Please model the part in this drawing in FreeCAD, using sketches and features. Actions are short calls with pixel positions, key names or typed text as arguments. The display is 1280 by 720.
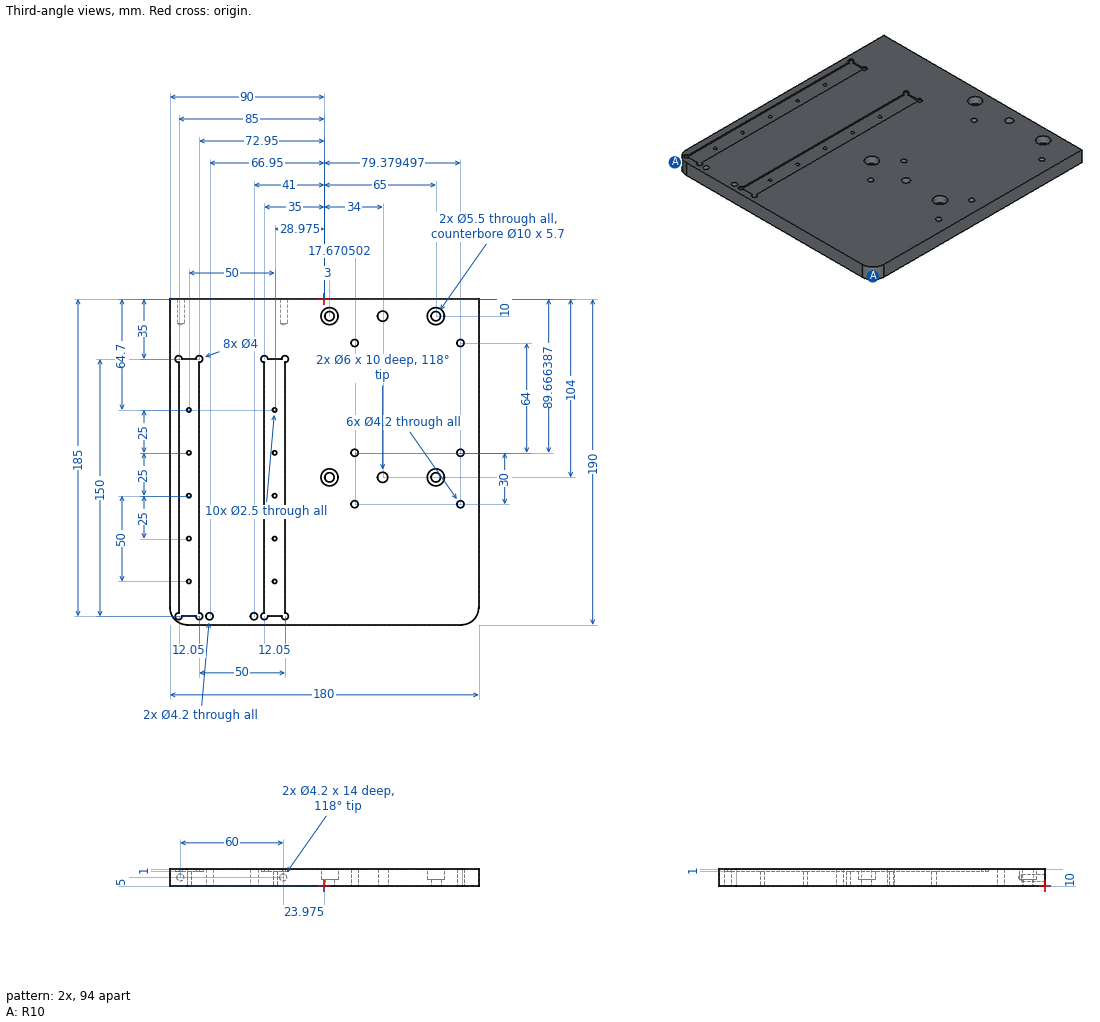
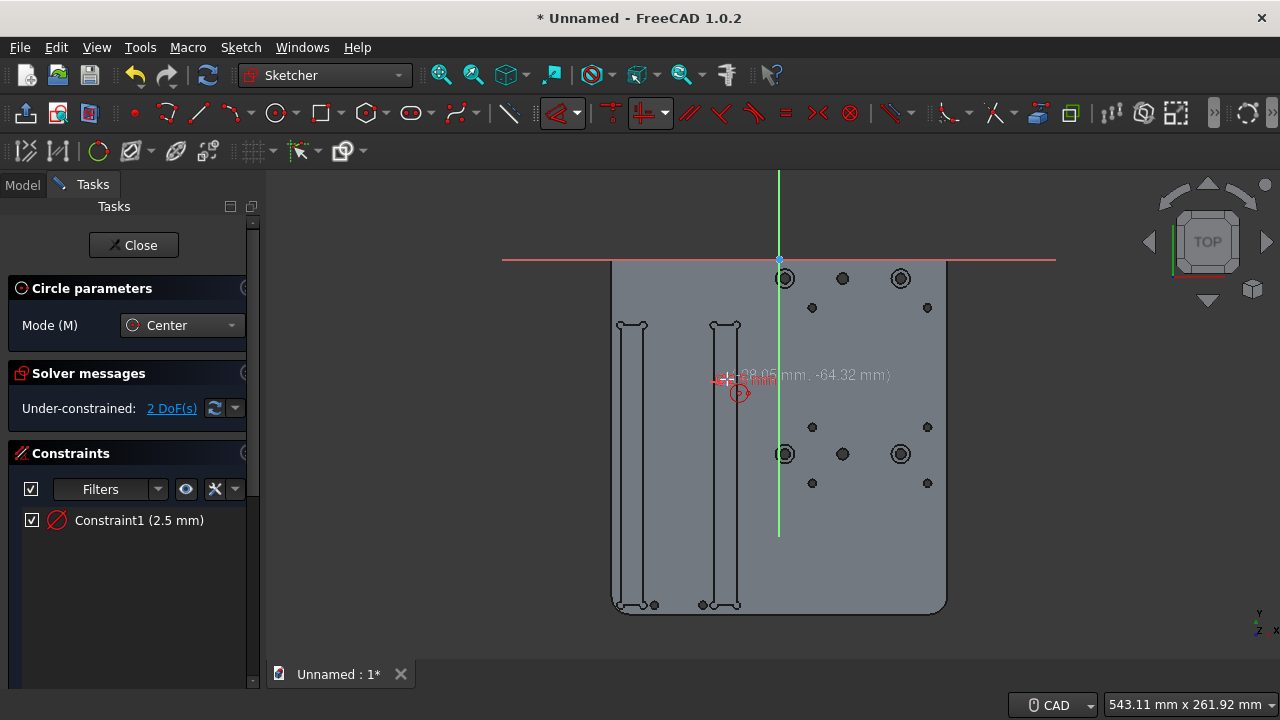
scroll(632, 381, up, 12)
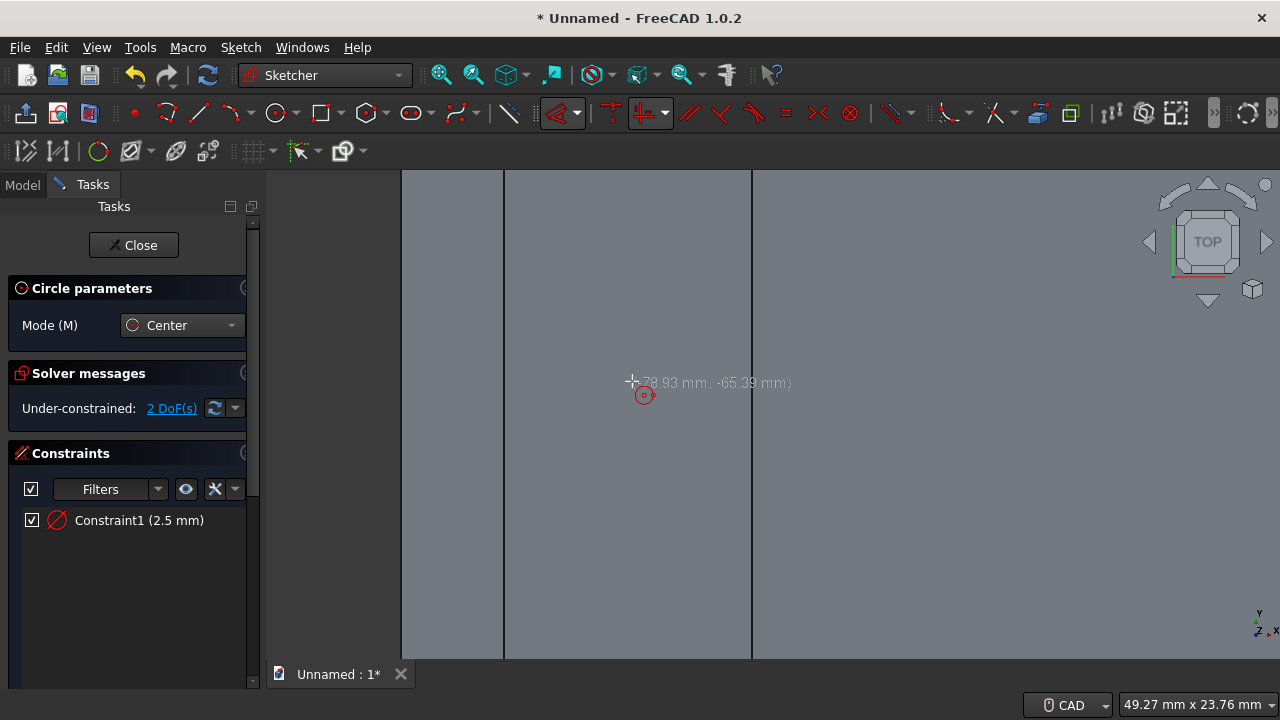
scroll(632, 381, down, 12)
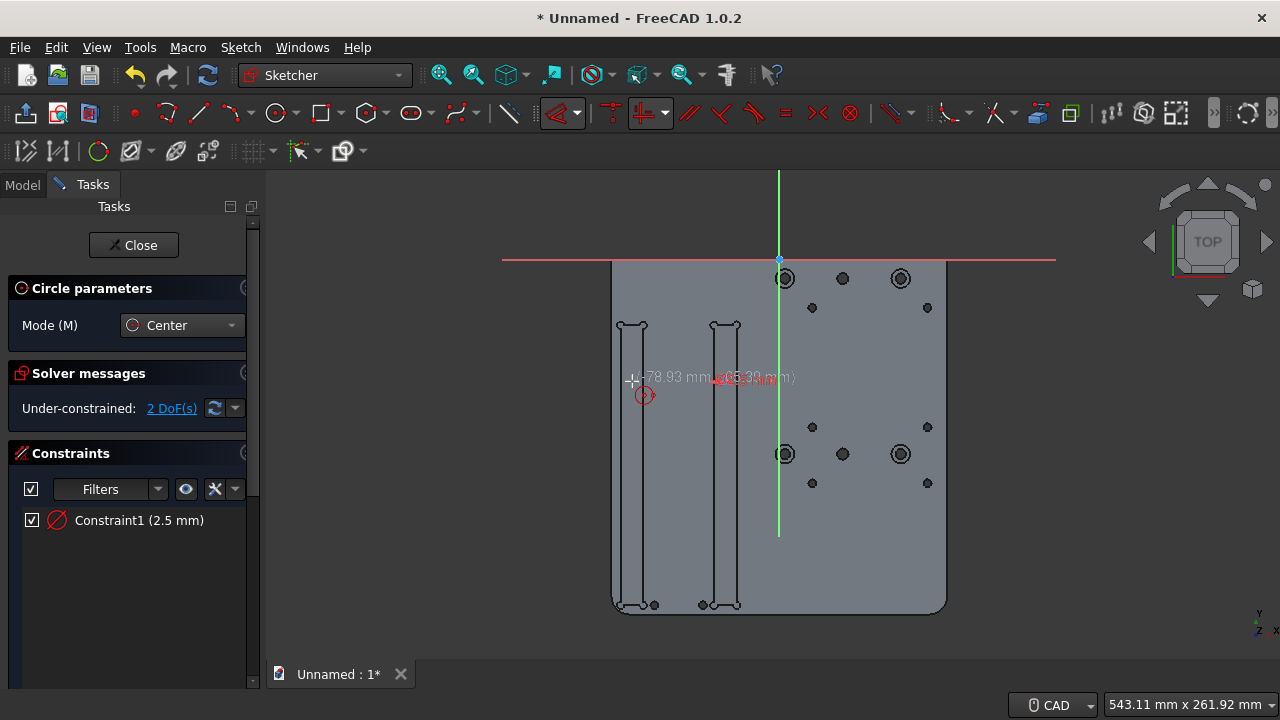
click(632, 381)
move(634, 379)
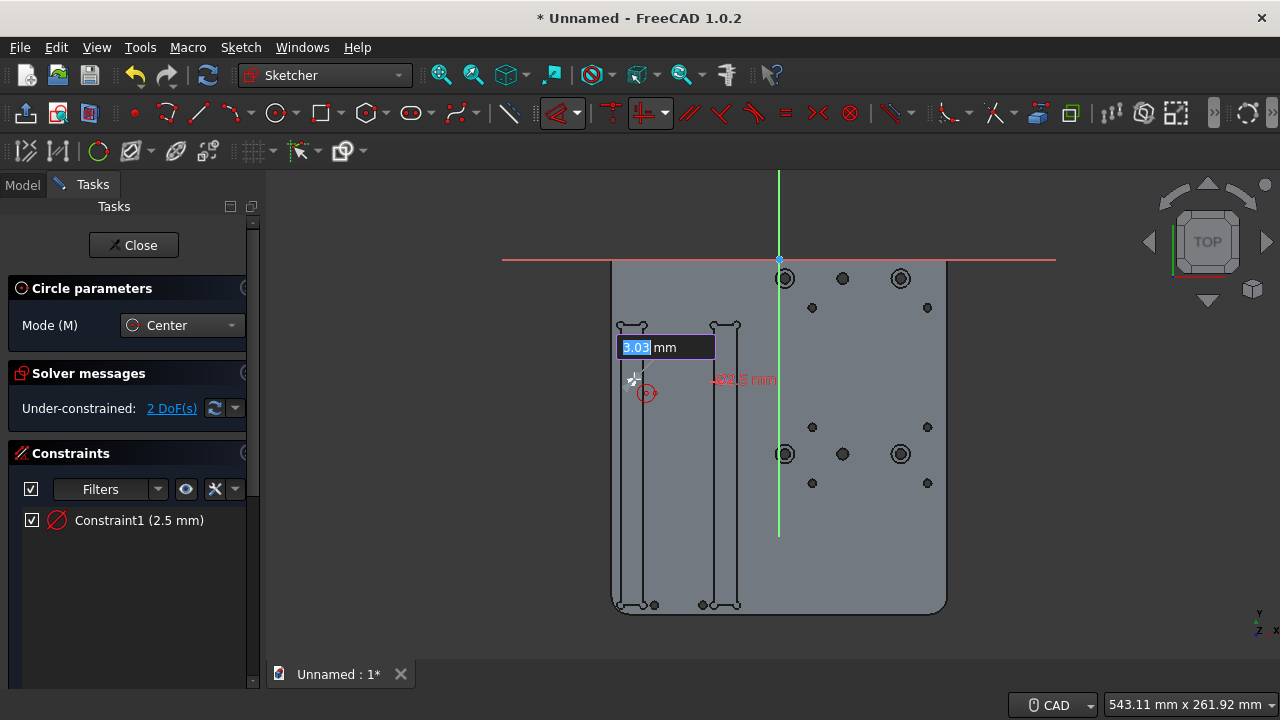
text(2.5)
key(Return)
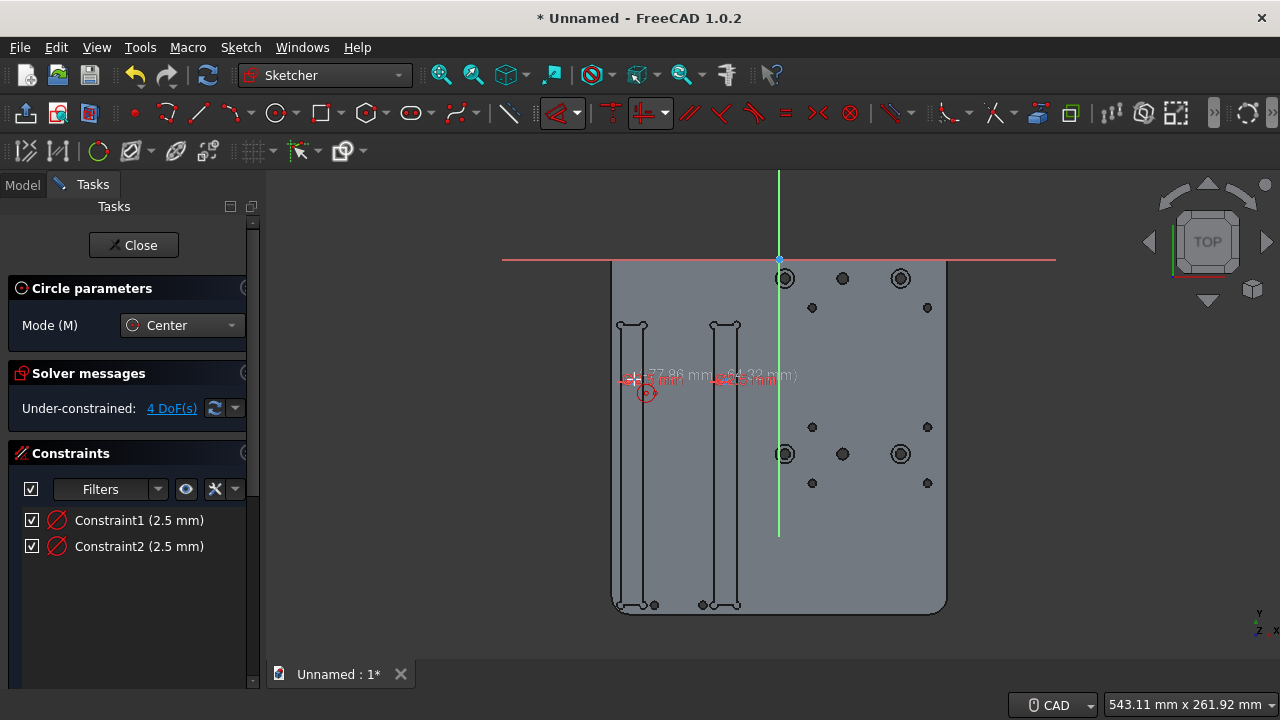
scroll(632, 427, up, 12)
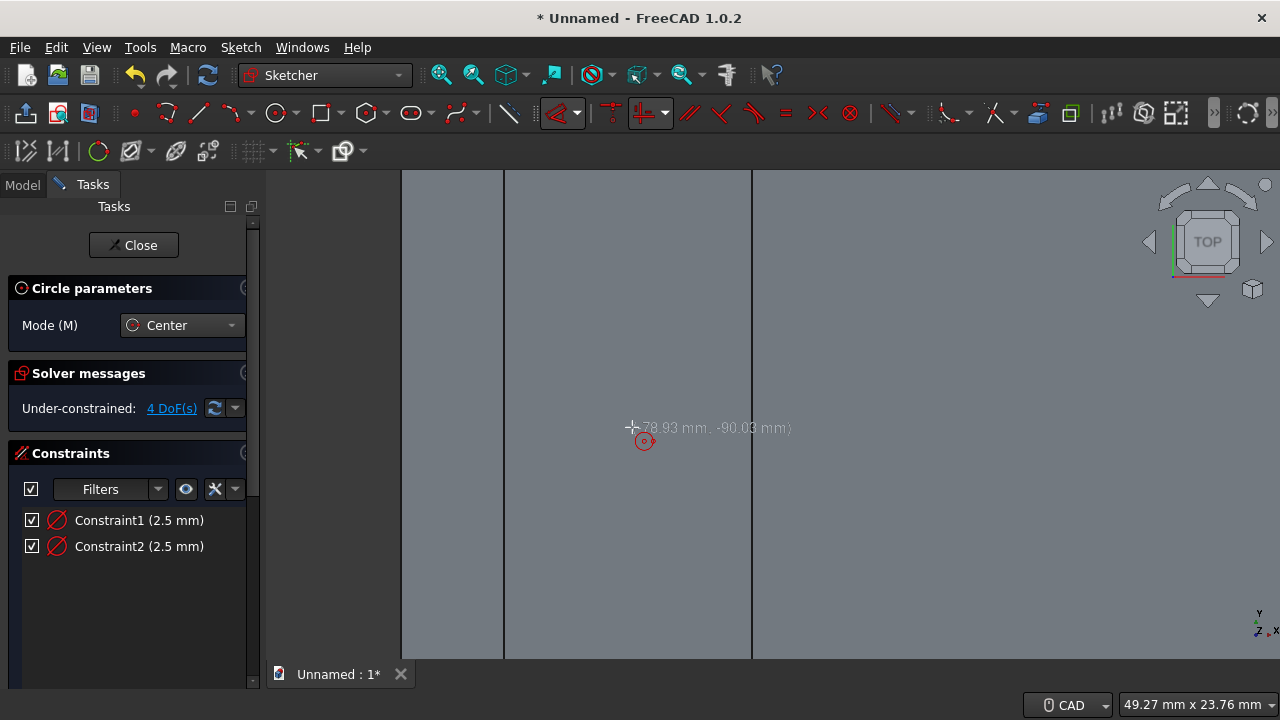
scroll(632, 427, down, 12)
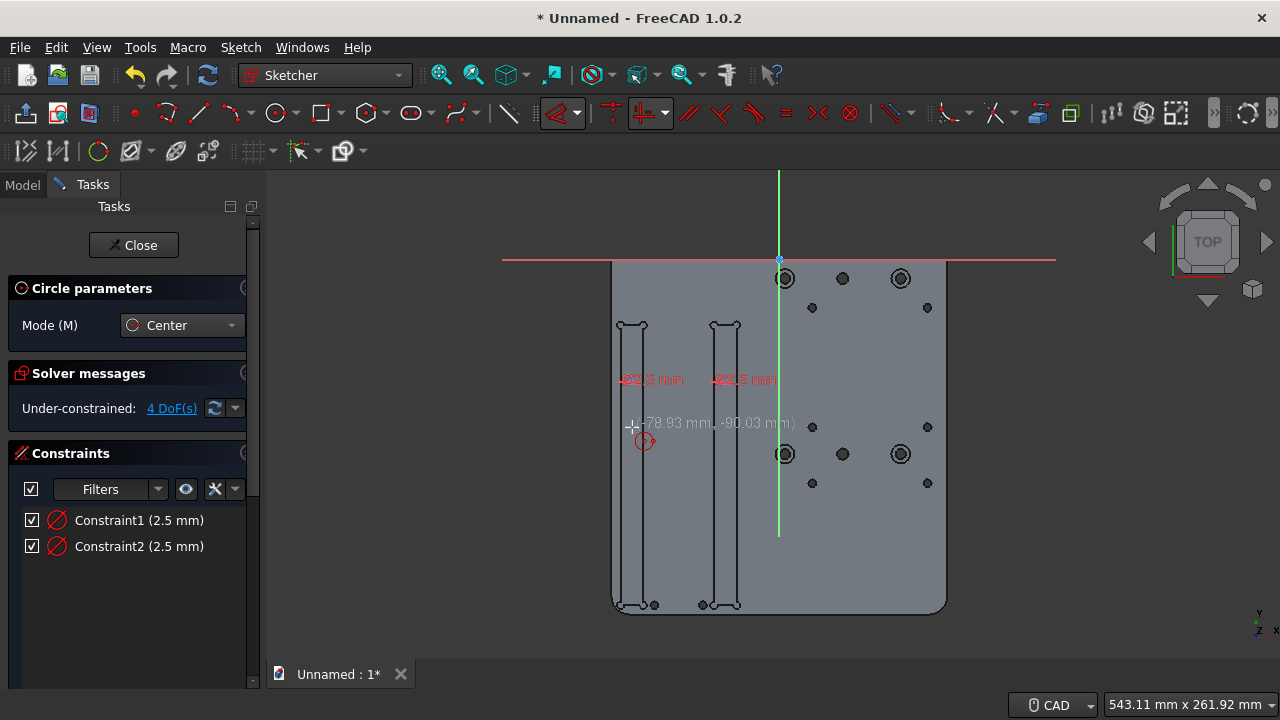
click(632, 427)
move(634, 426)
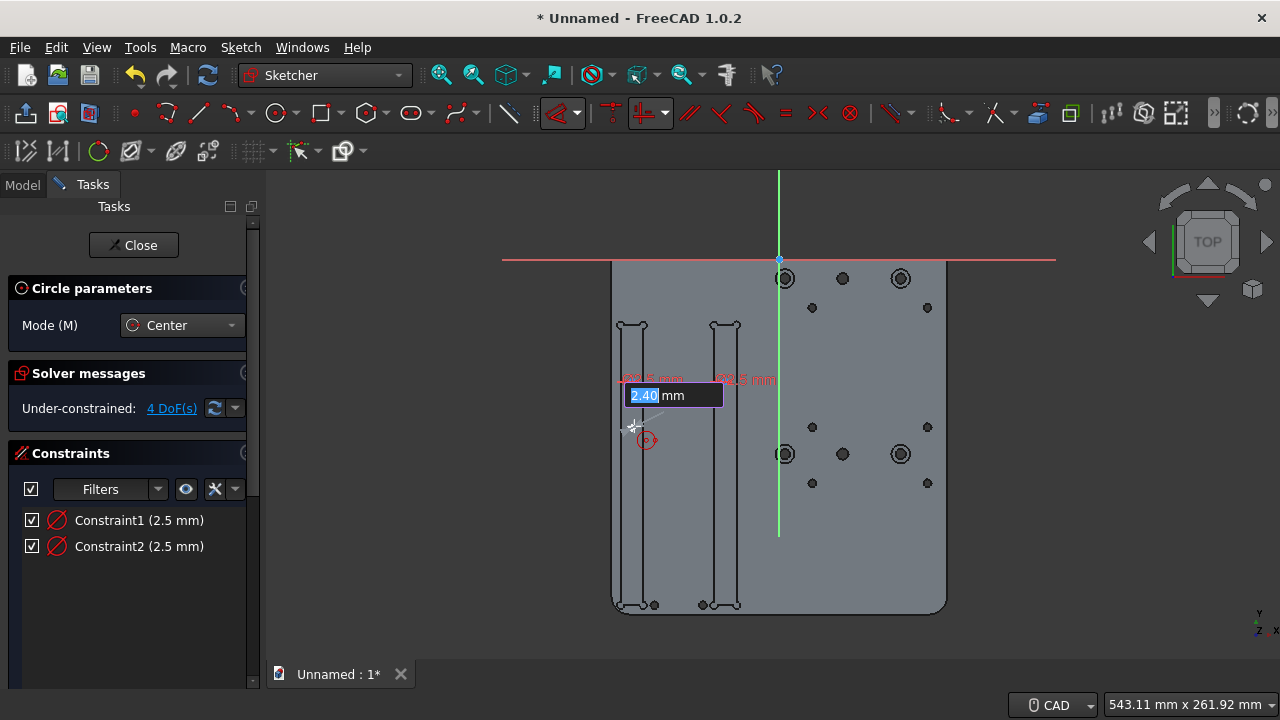
text(2.5)
key(Return)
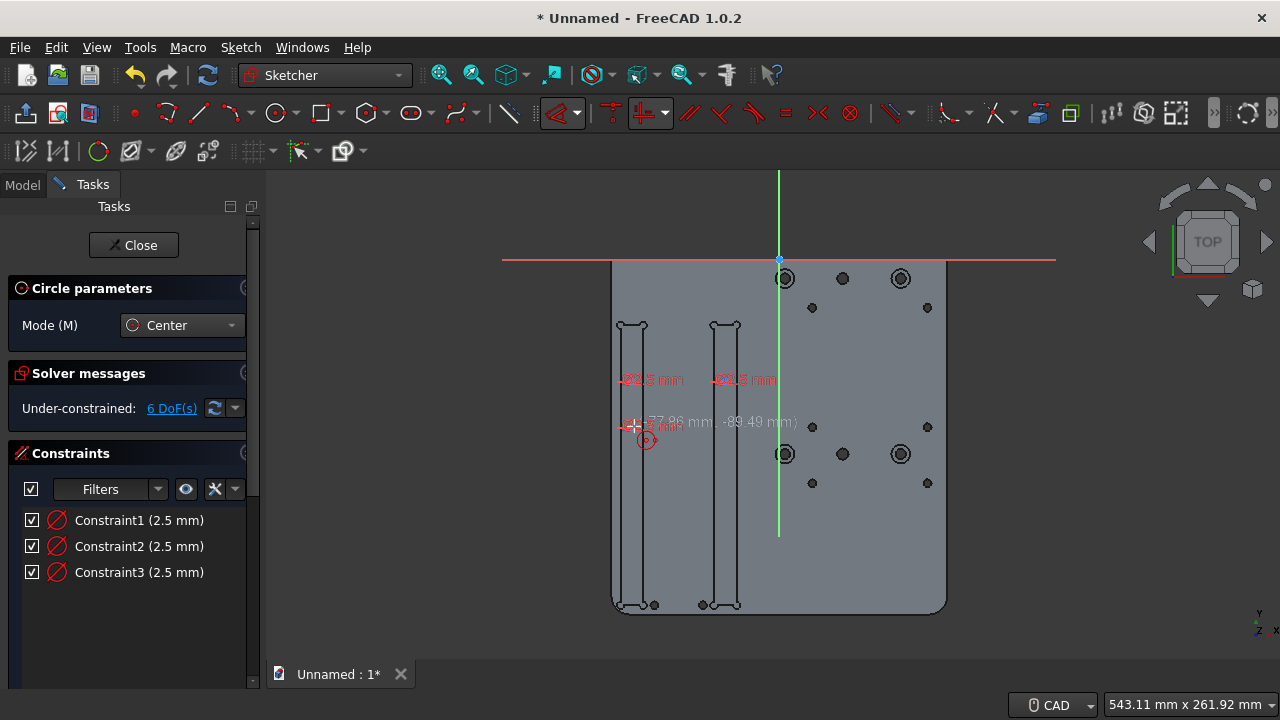
scroll(632, 474, up, 12)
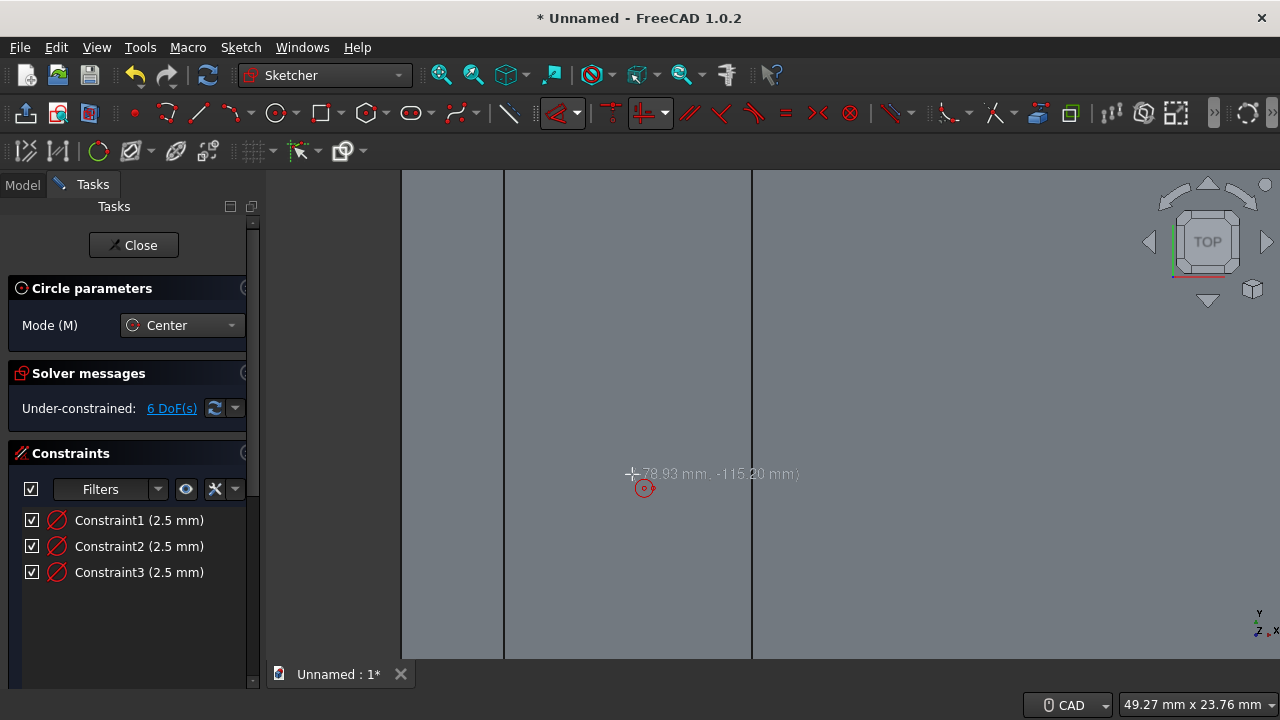
scroll(632, 474, down, 12)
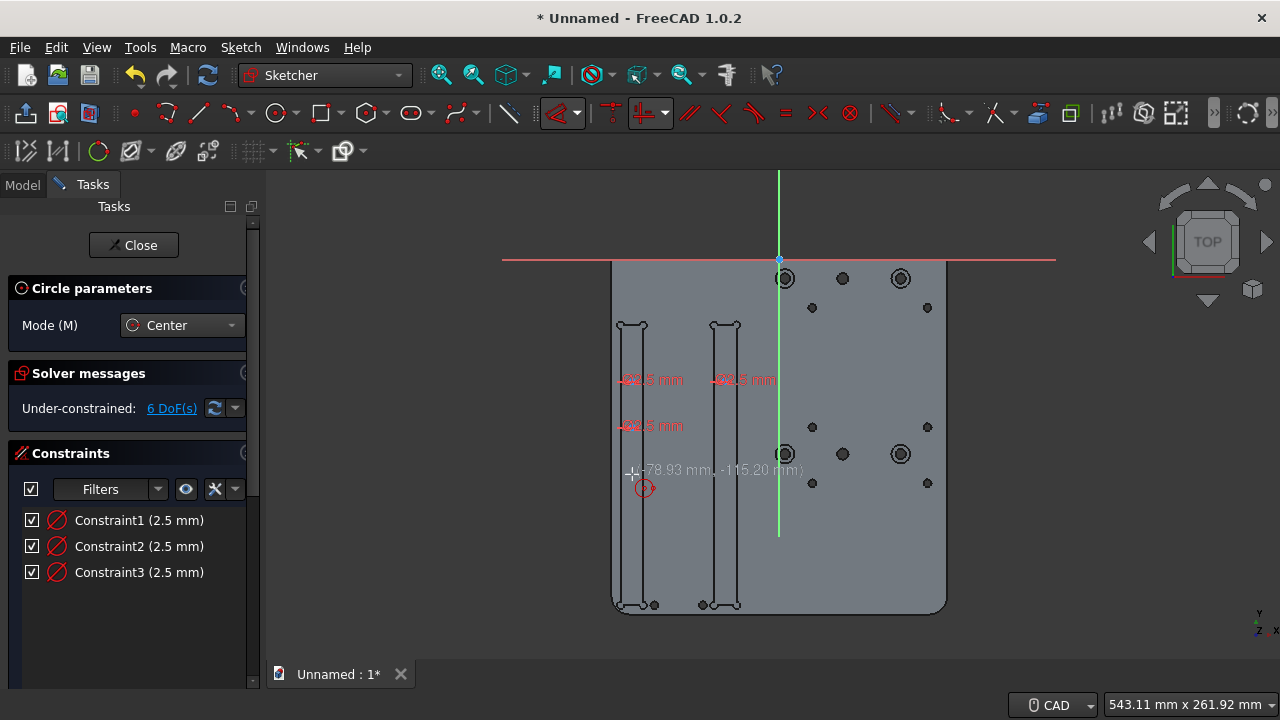
click(632, 474)
move(634, 472)